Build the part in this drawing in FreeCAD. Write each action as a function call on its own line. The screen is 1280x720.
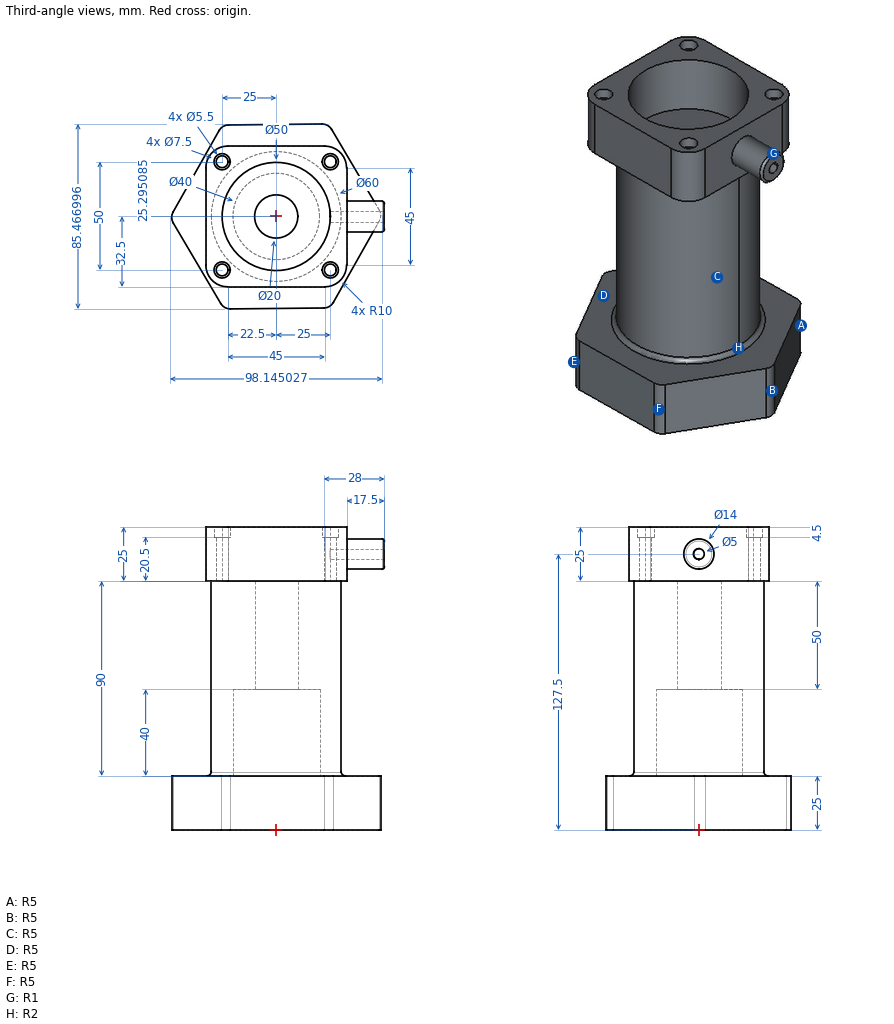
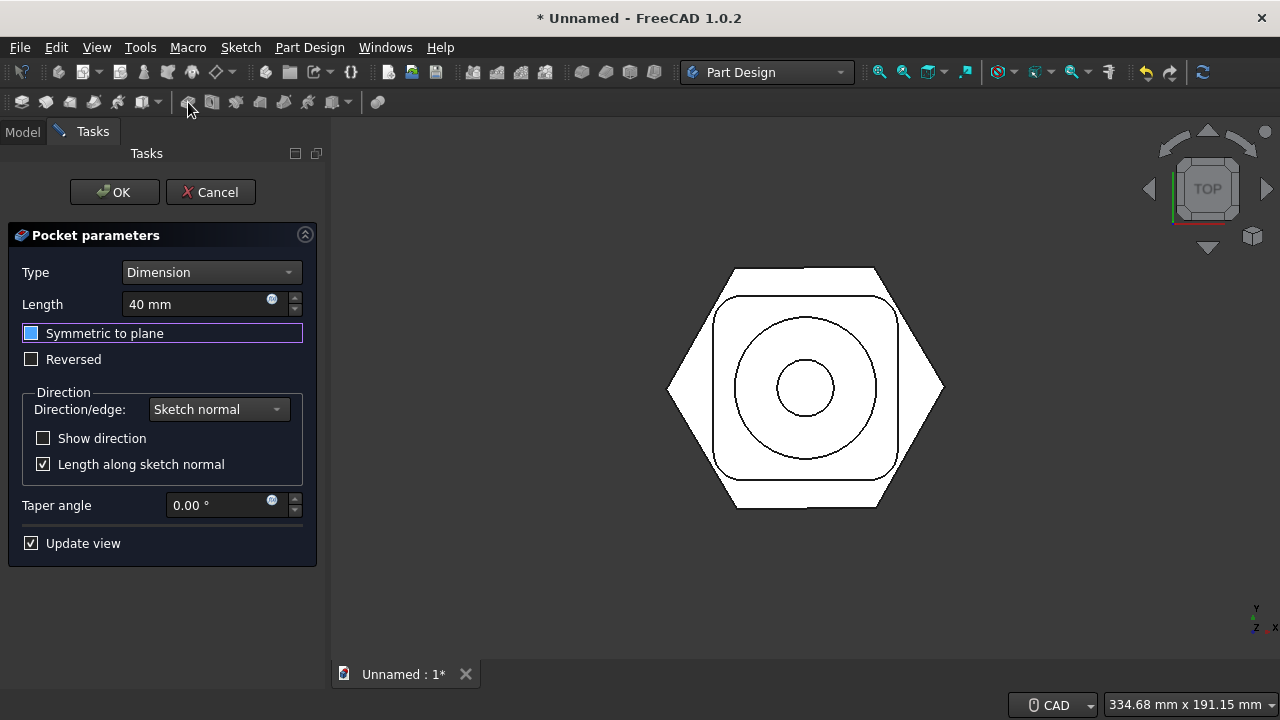
click(115, 192)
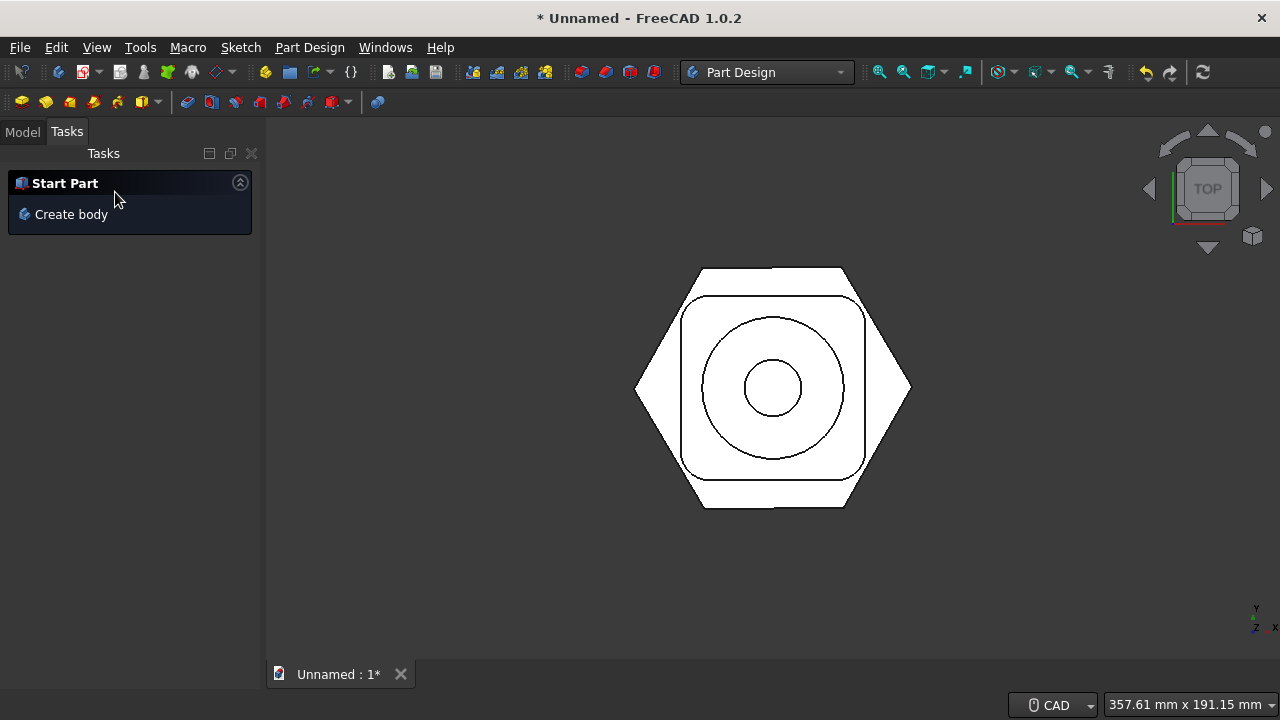
click(880, 72)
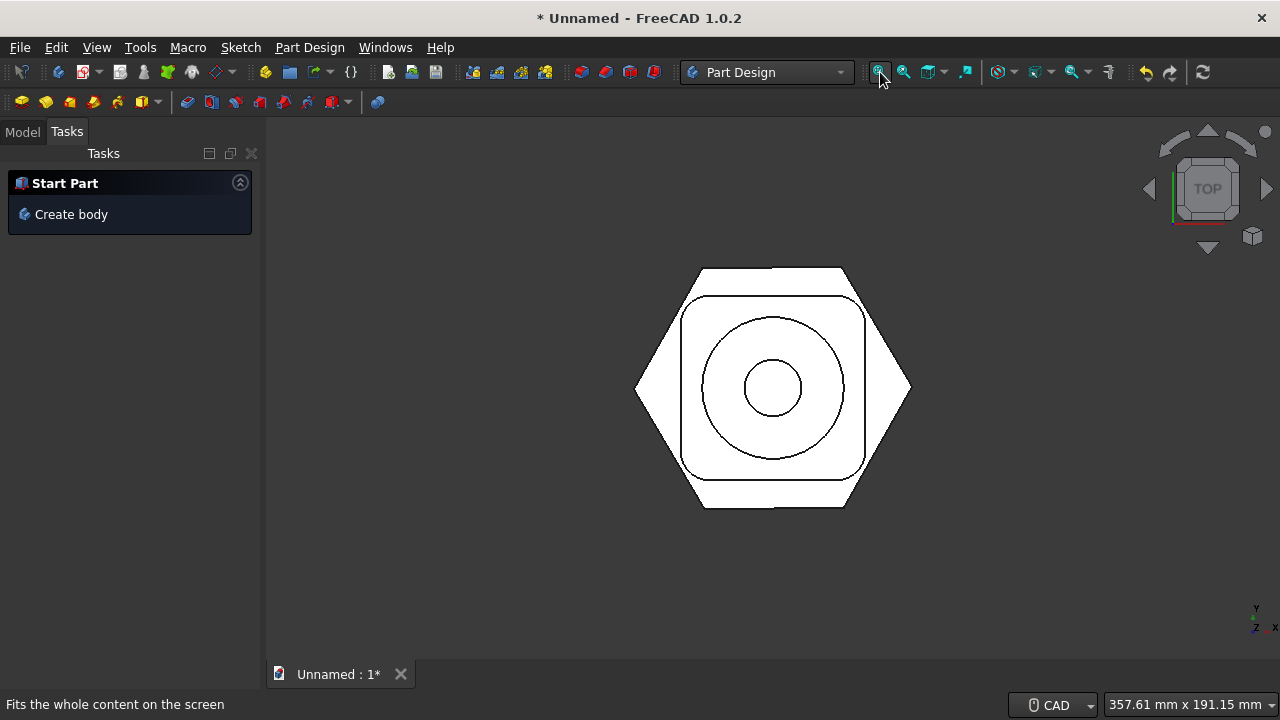
key(0)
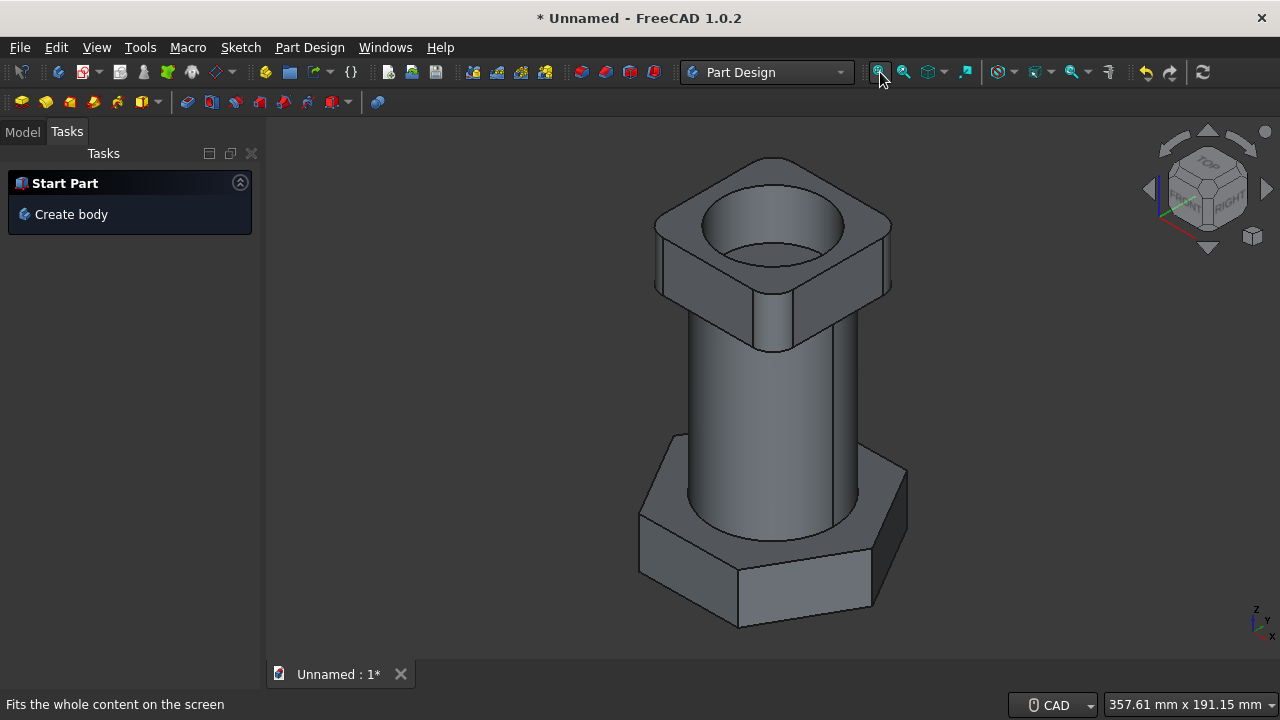
key(2)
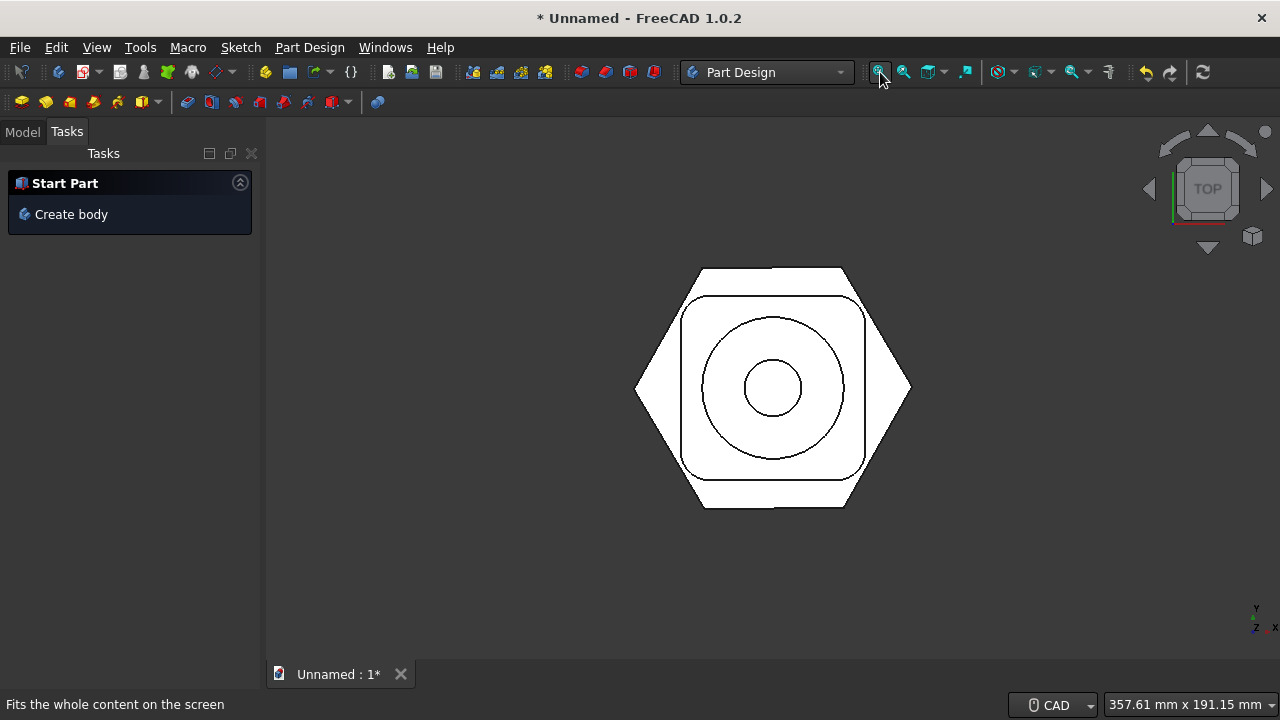
click(880, 72)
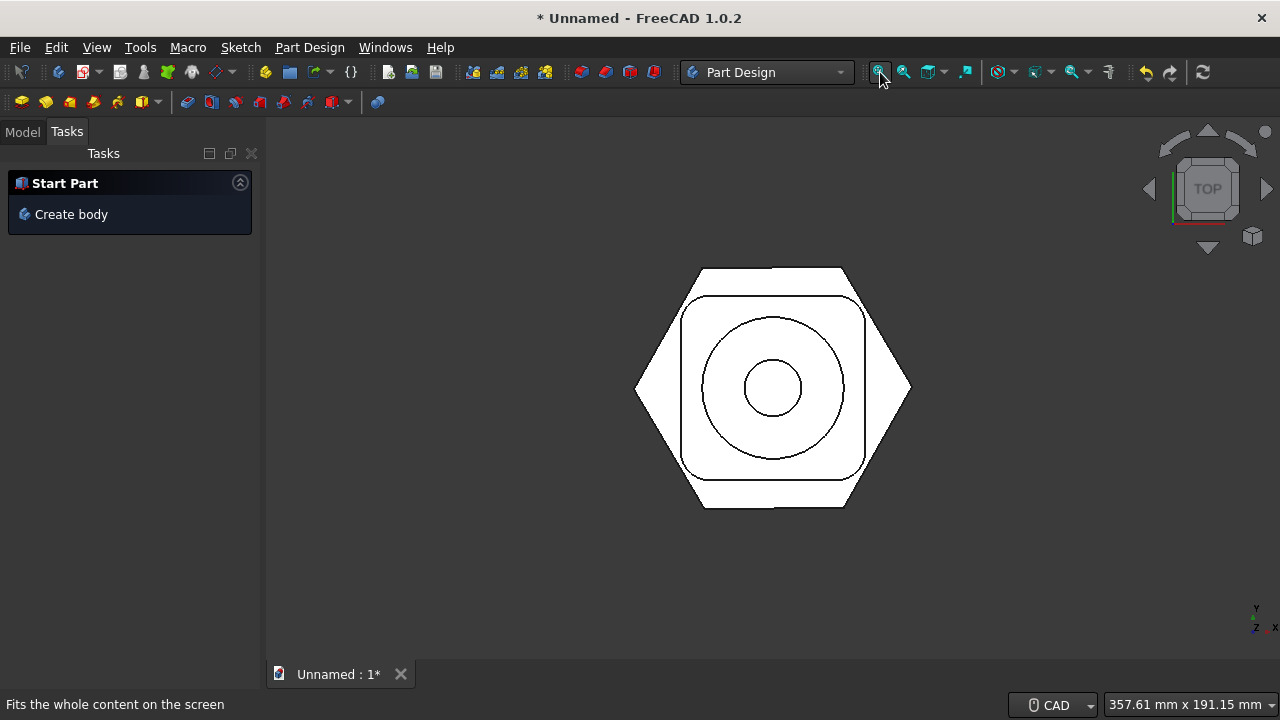
key(1)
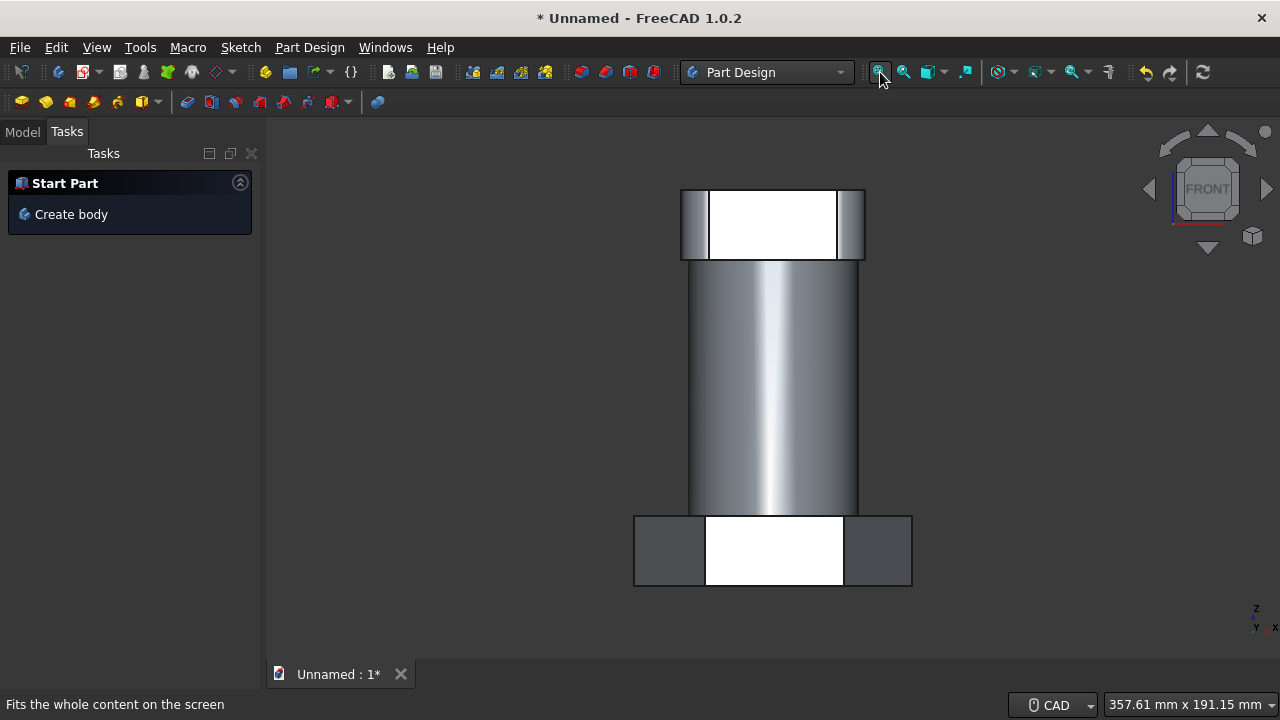
key(3)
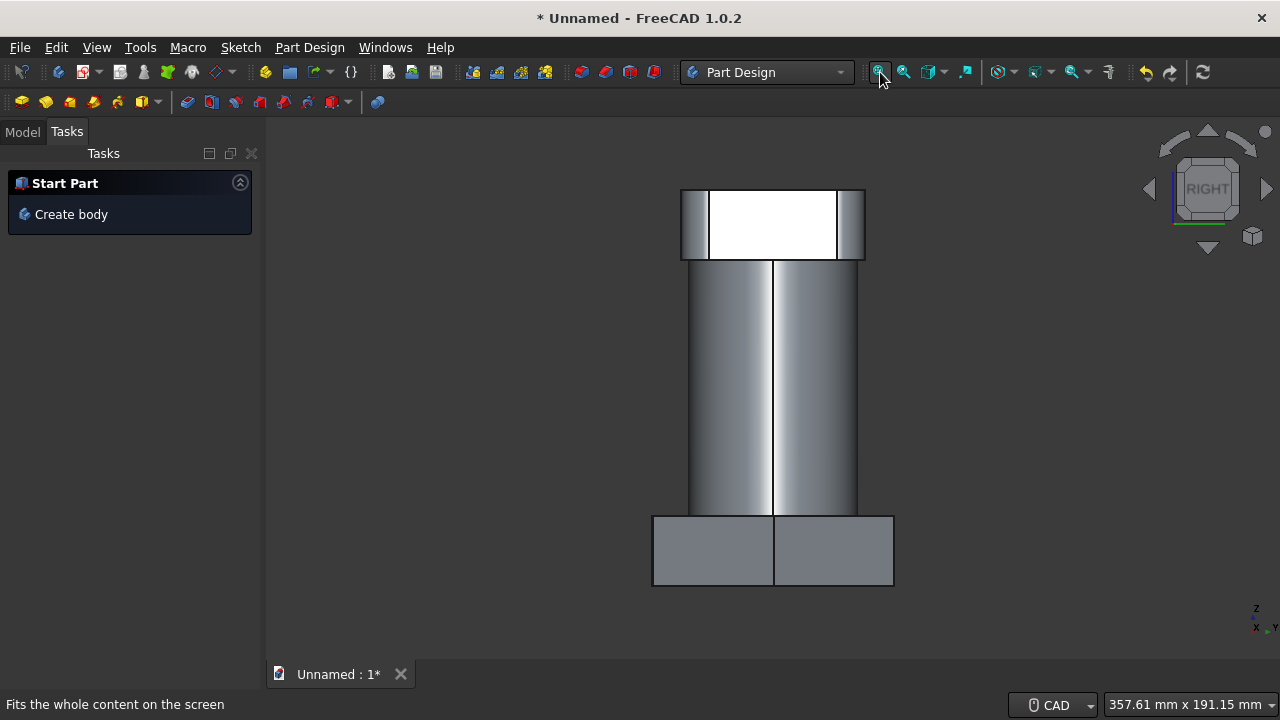
key(5)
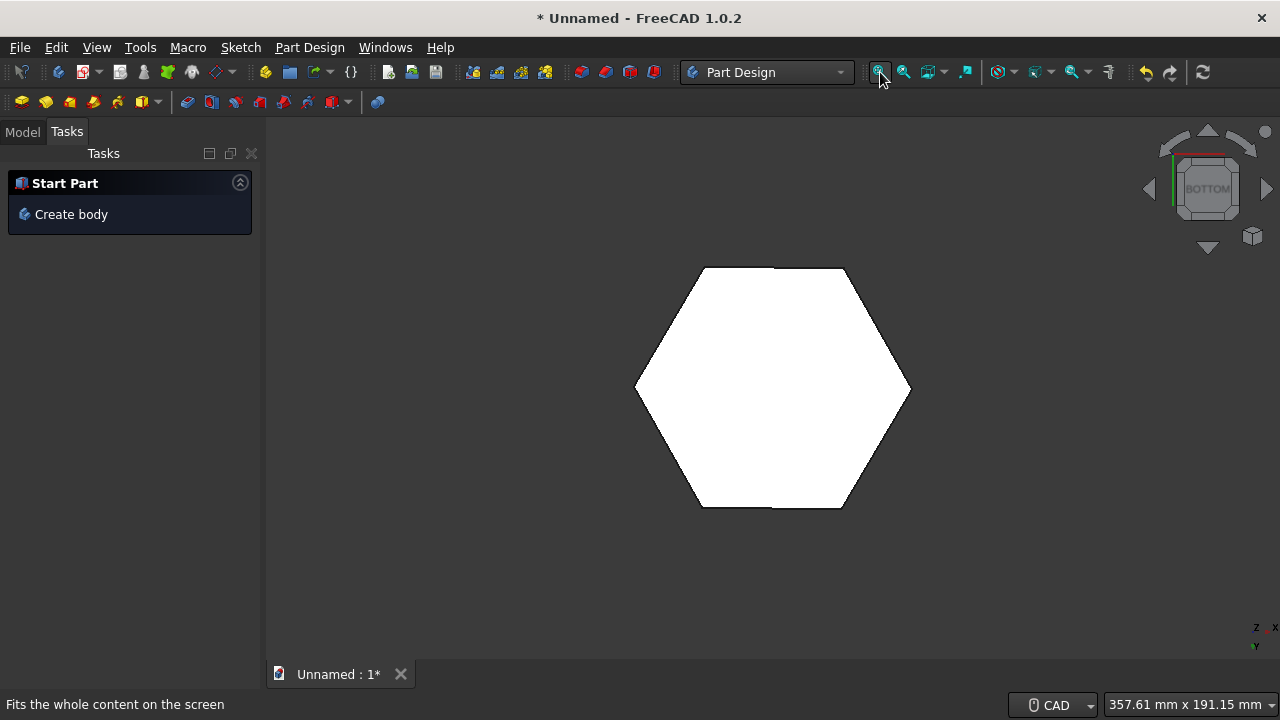
click(880, 72)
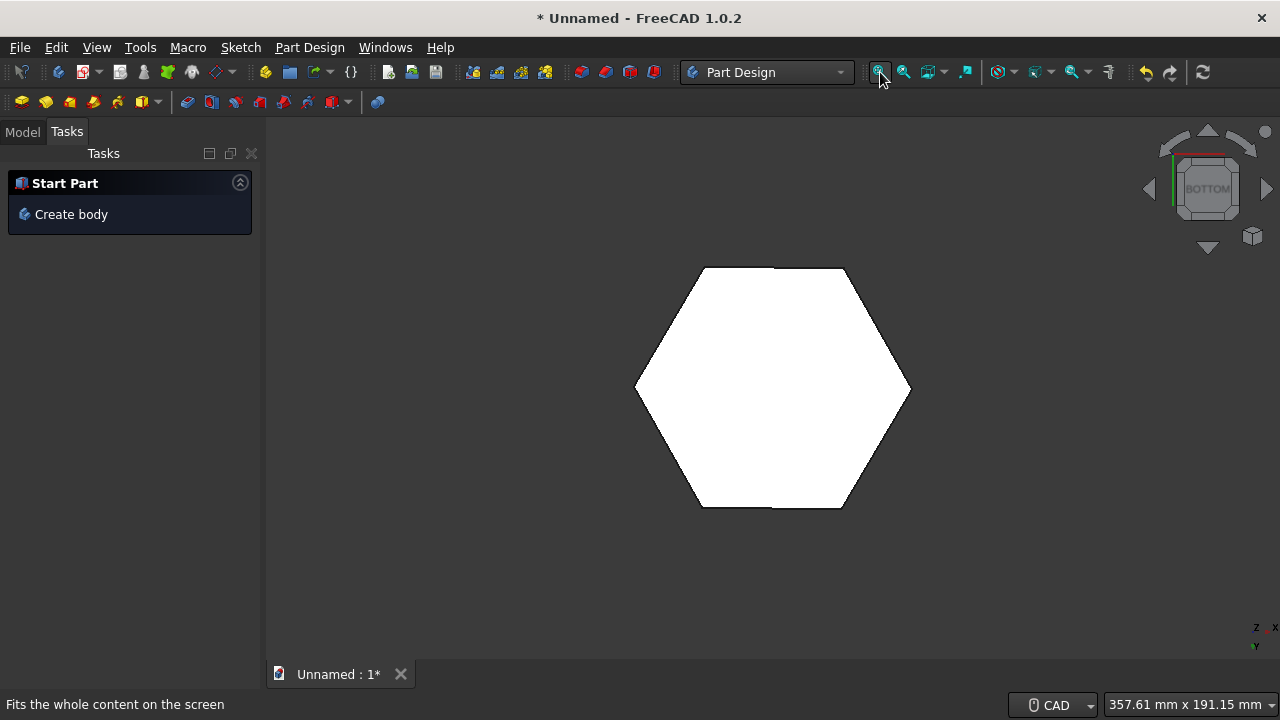
key(4)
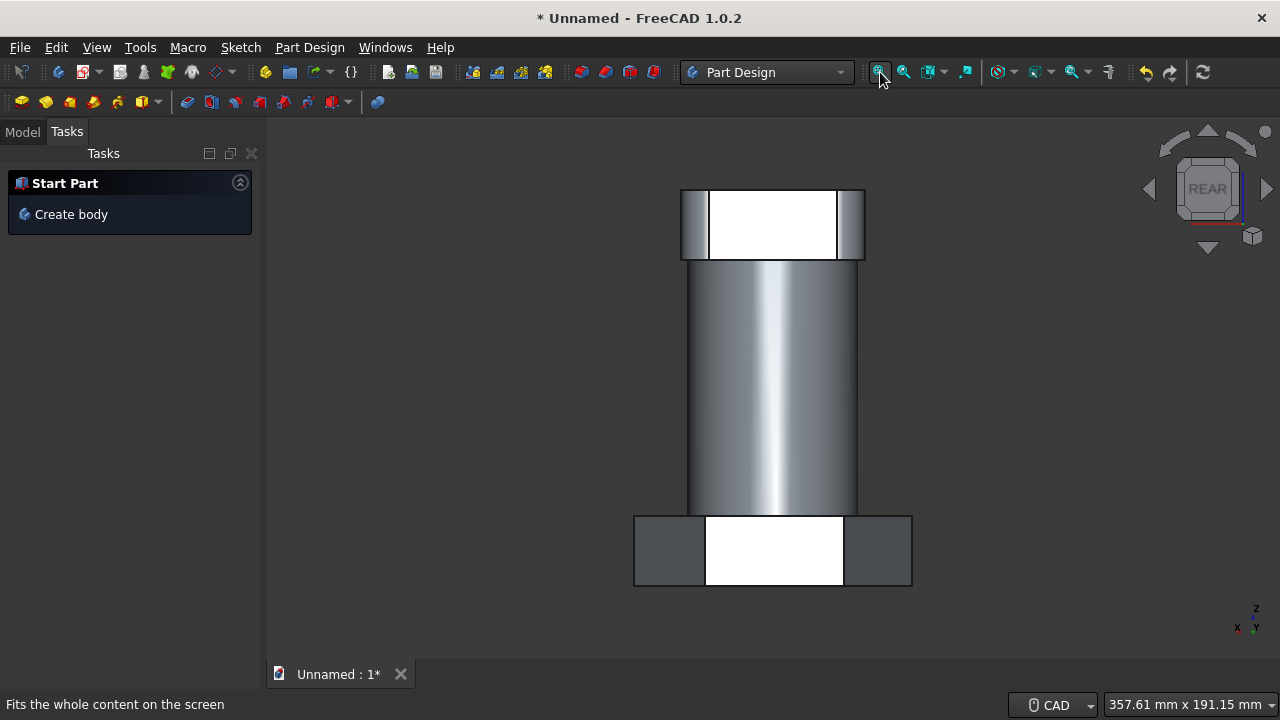
click(705, 550)